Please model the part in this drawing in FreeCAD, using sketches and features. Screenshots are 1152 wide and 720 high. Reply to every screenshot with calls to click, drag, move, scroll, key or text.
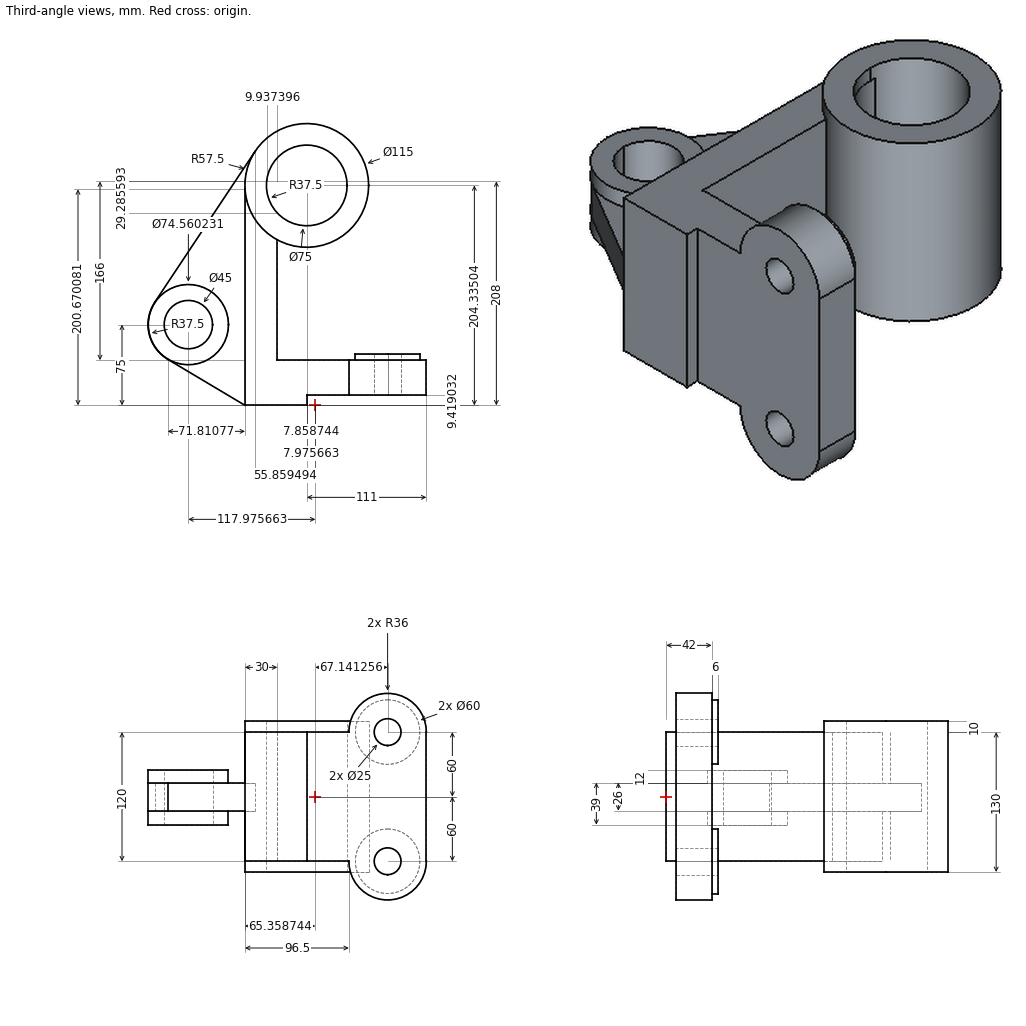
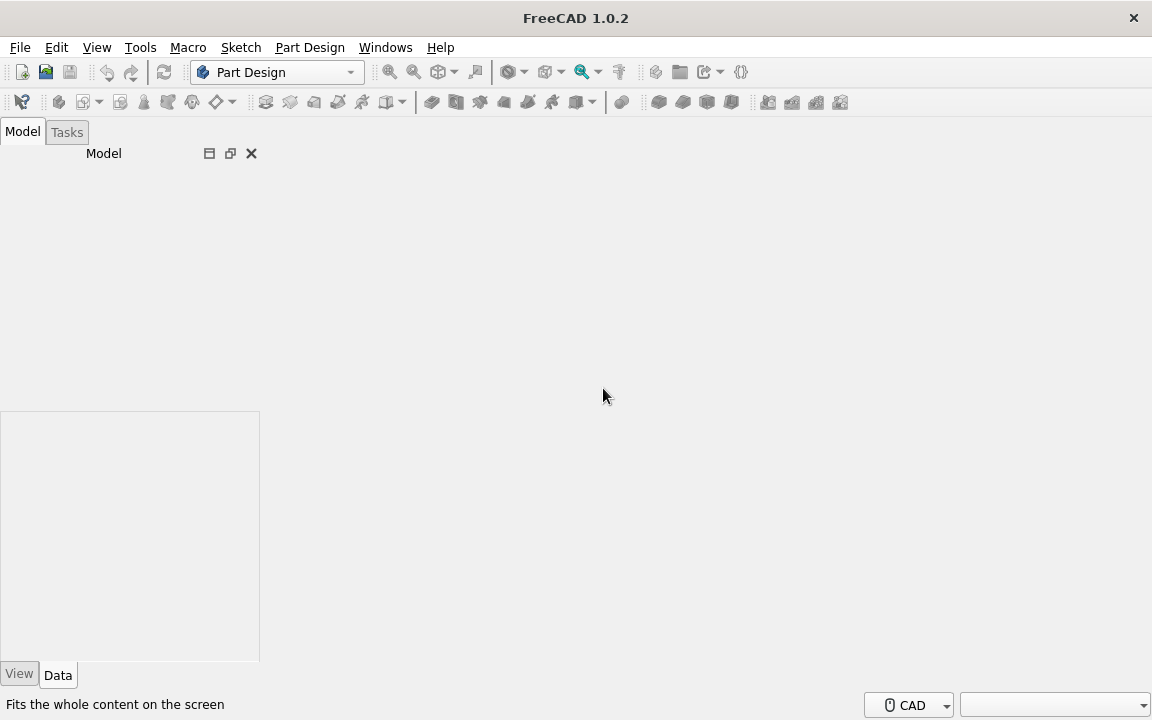
click(22, 72)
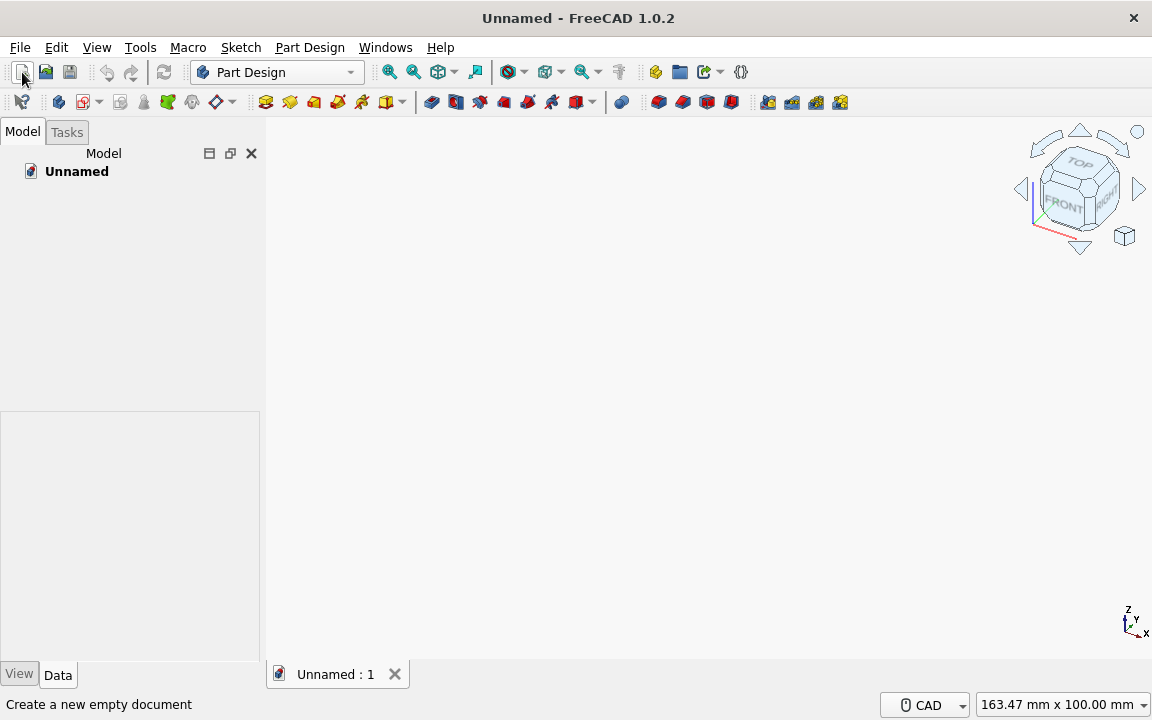
click(84, 102)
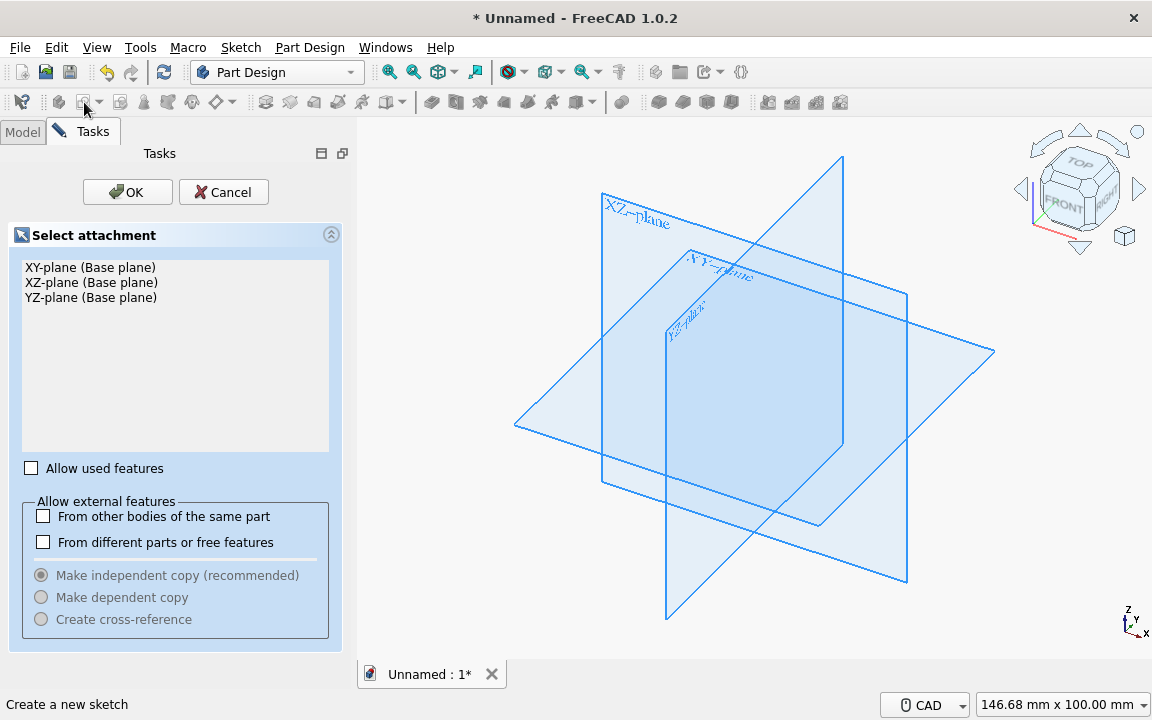
click(82, 282)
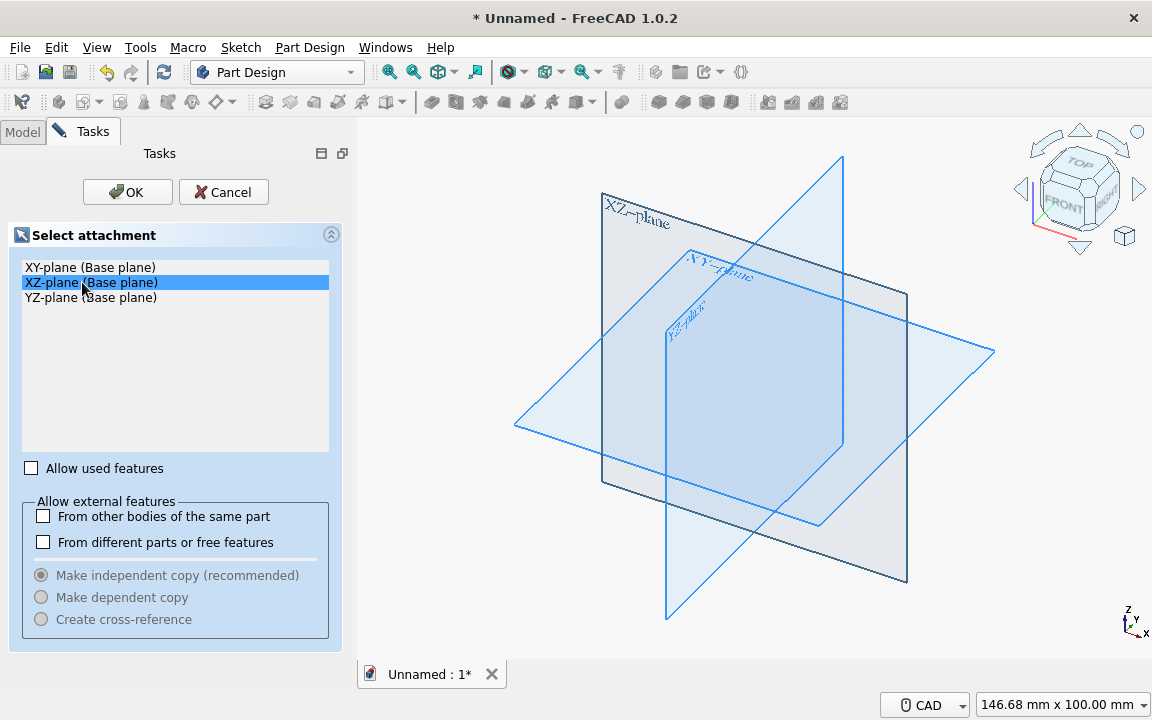
click(128, 192)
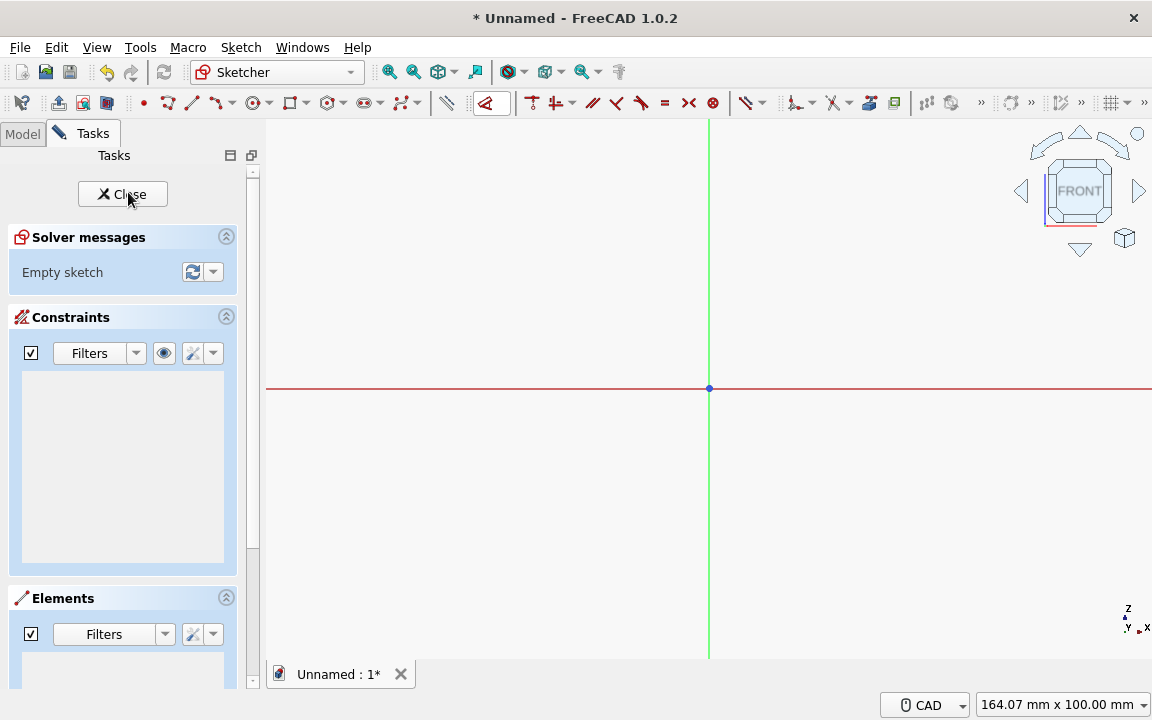
scroll(567, 389, down, 6)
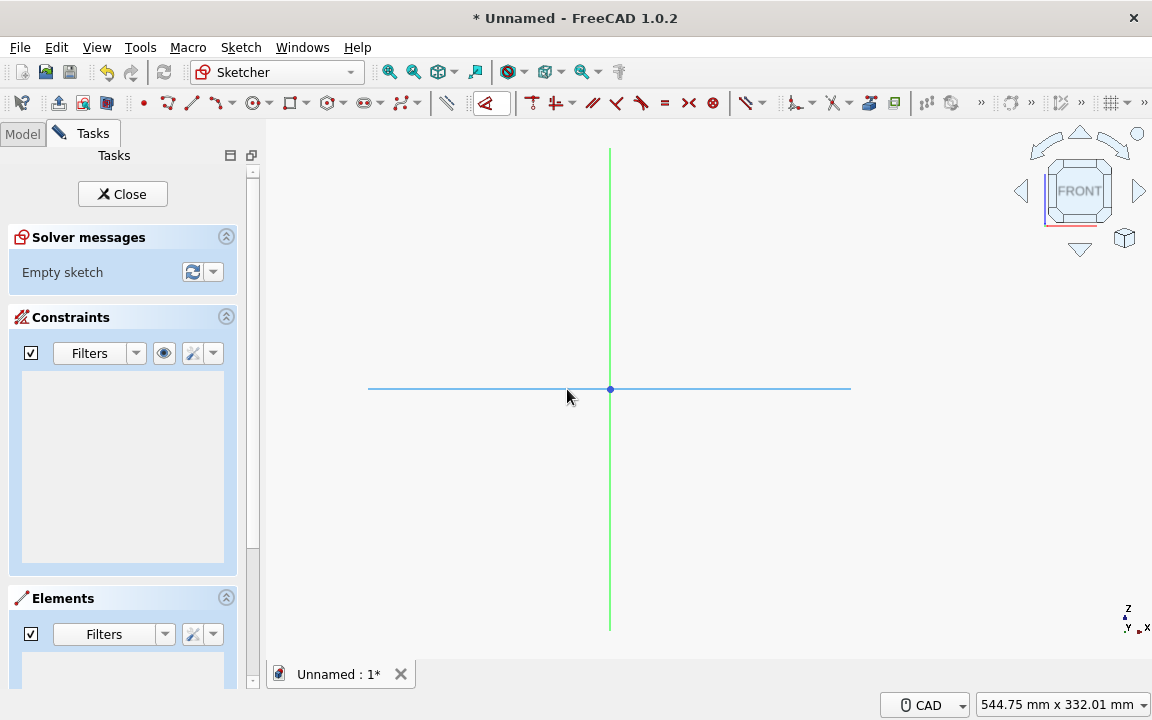
click(168, 104)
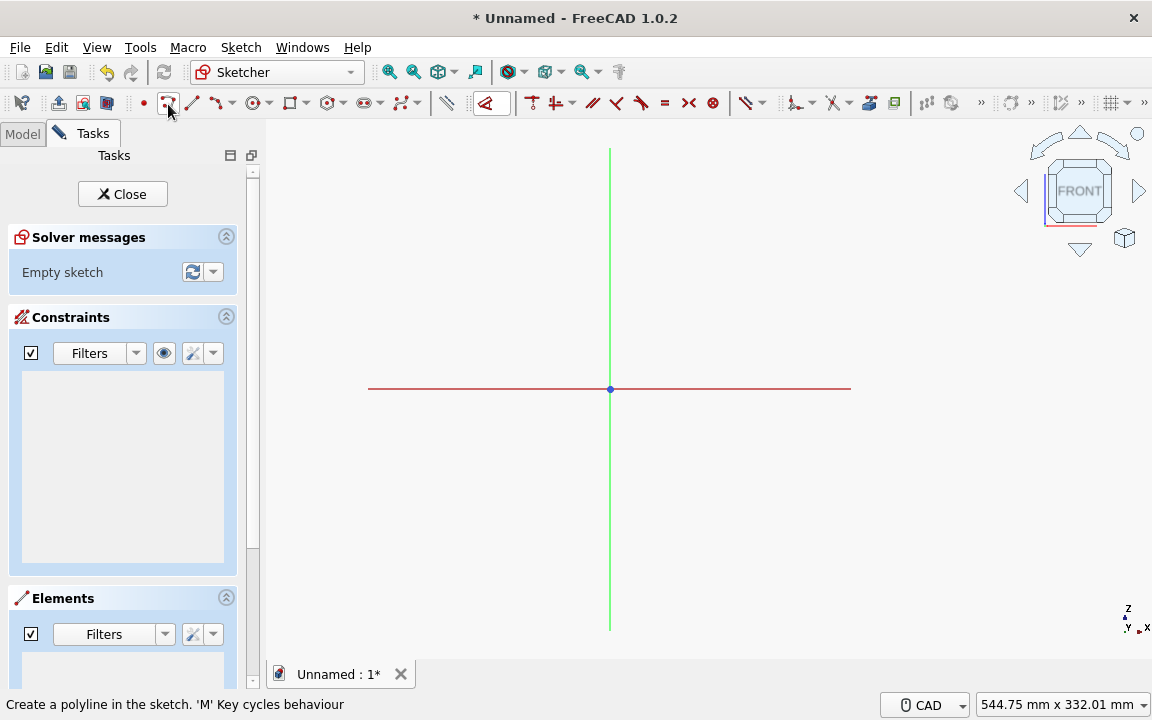
click(661, 487)
click(504, 487)
click(504, 292)
click(661, 292)
right_click(661, 292)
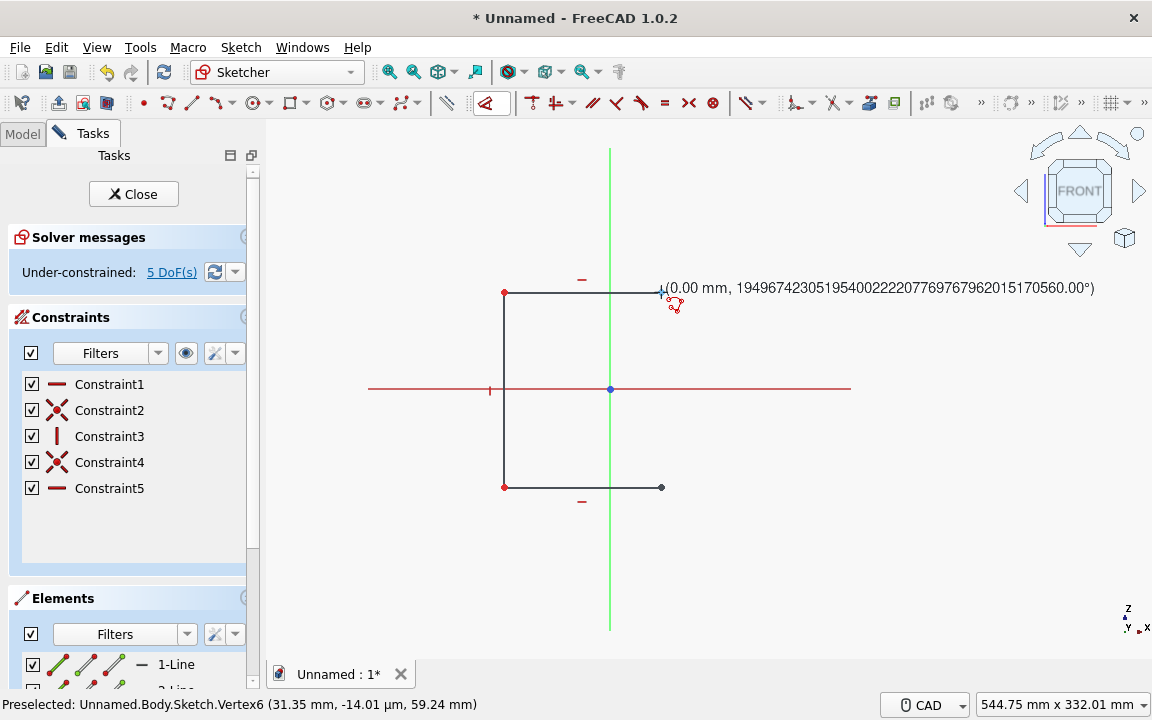
click(192, 104)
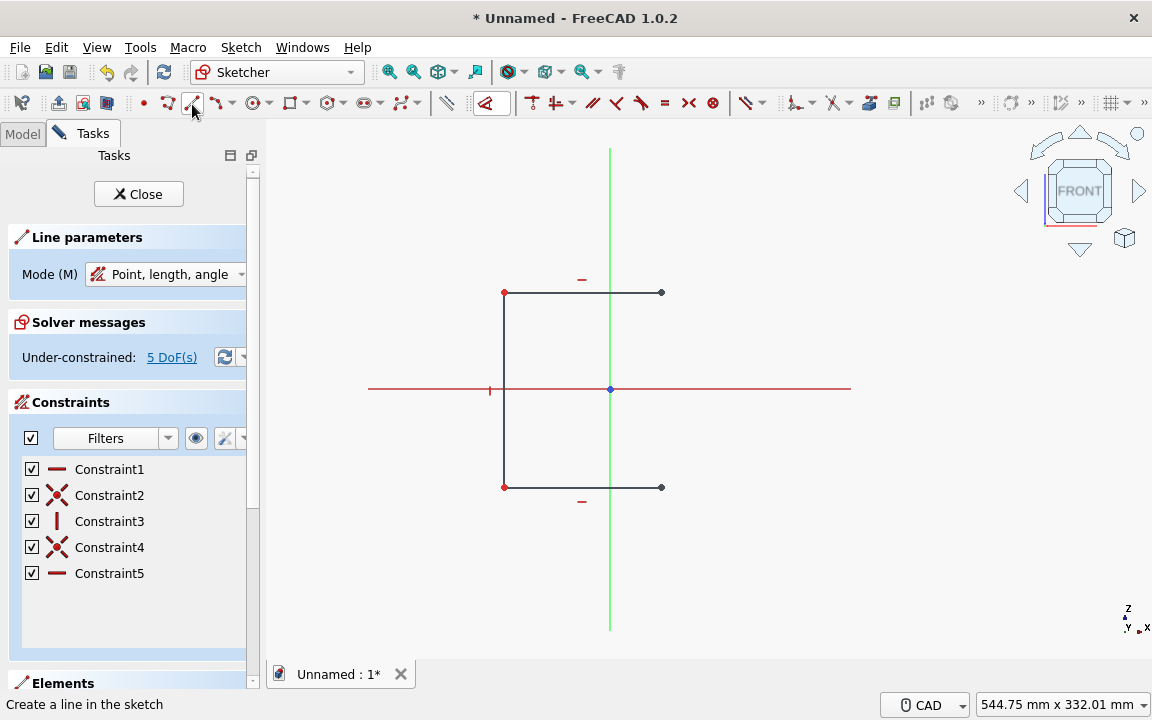
click(778, 292)
click(778, 487)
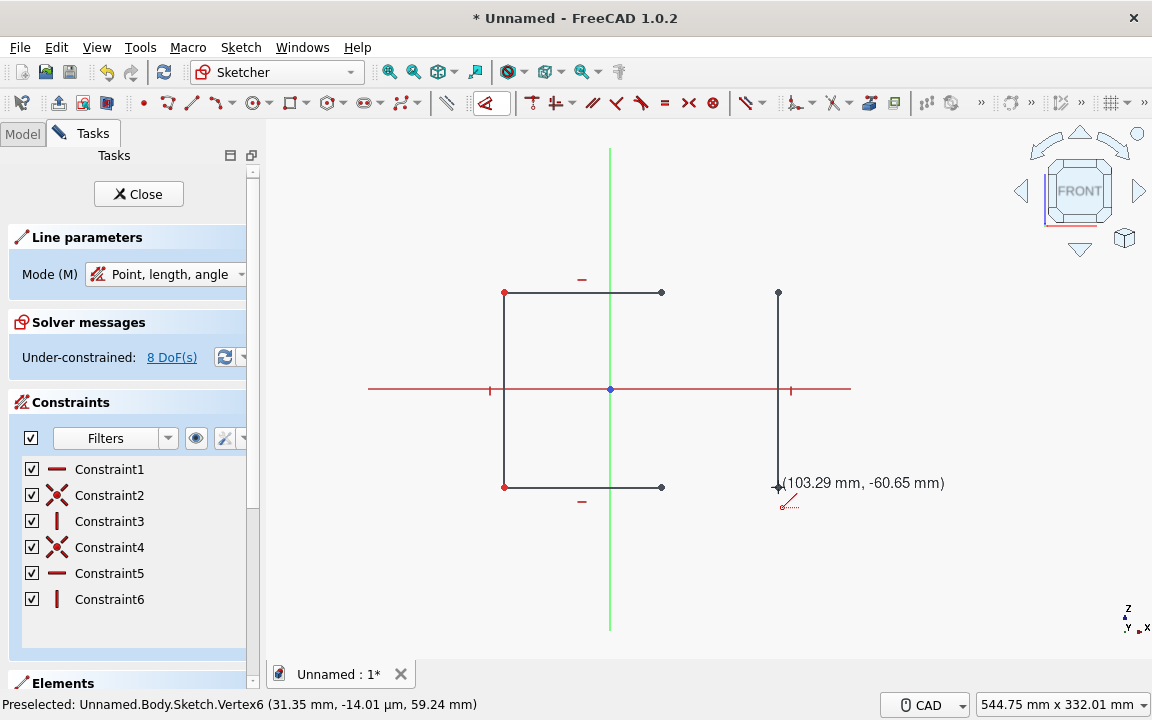
click(216, 104)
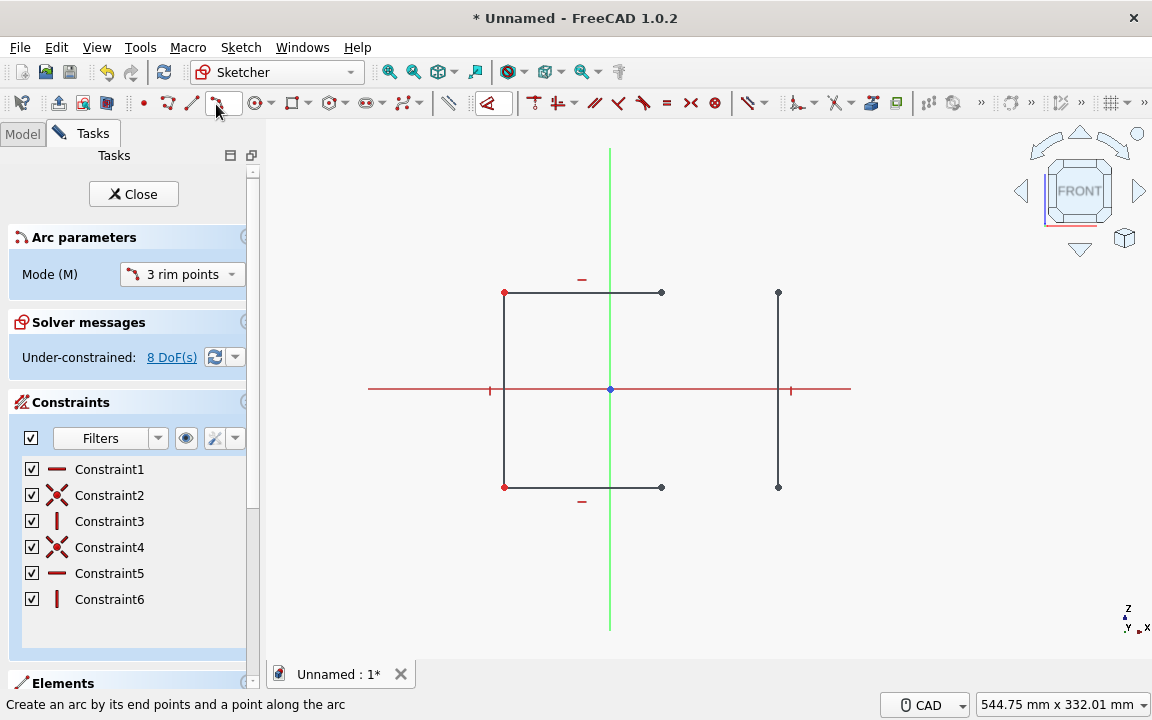
click(661, 293)
click(778, 293)
click(719, 233)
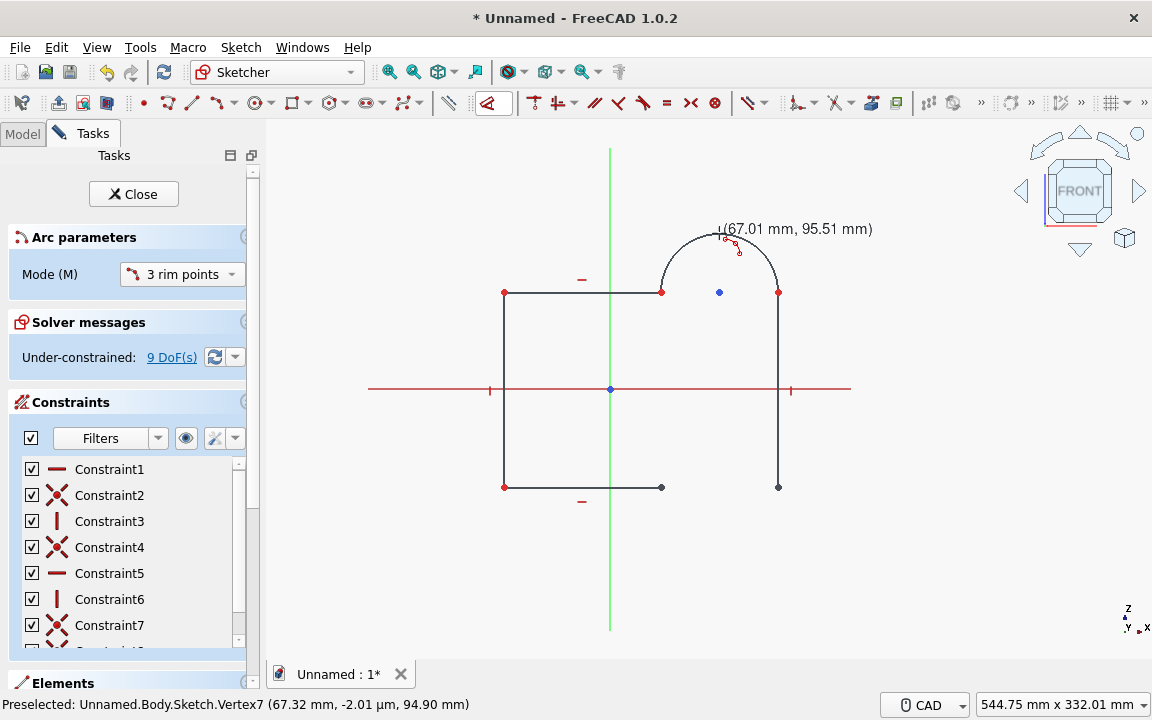
click(778, 488)
click(661, 488)
click(719, 545)